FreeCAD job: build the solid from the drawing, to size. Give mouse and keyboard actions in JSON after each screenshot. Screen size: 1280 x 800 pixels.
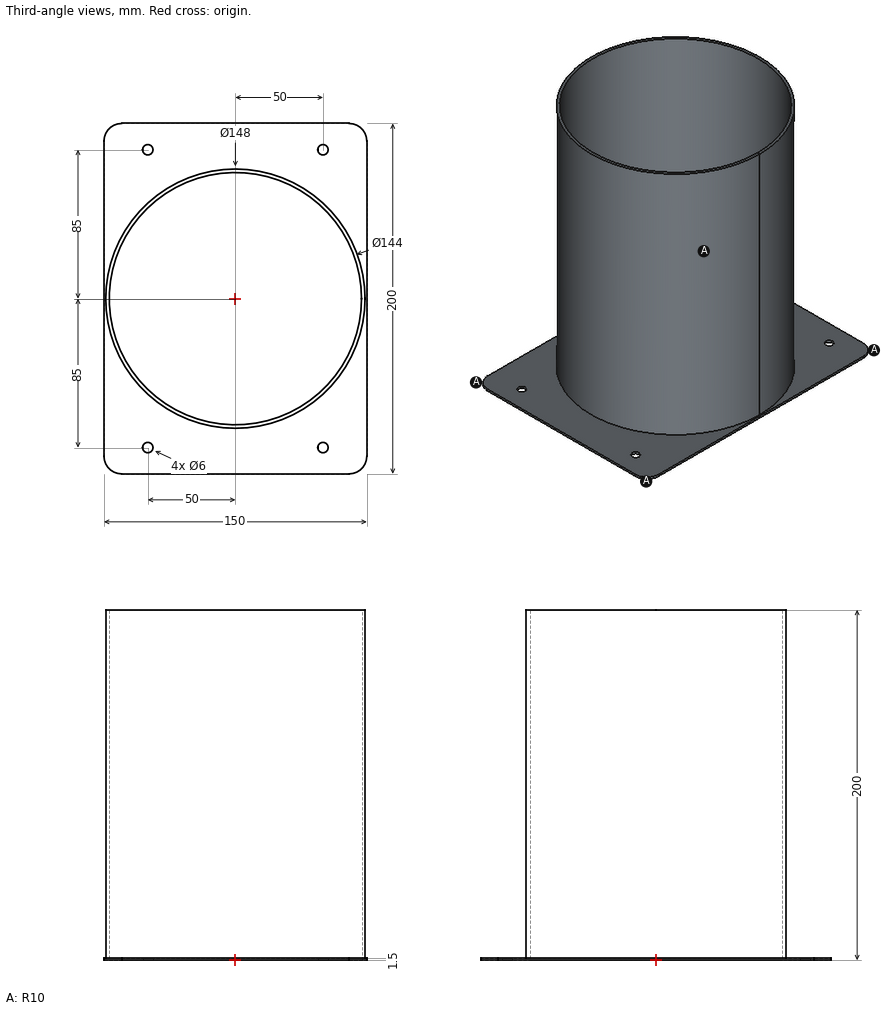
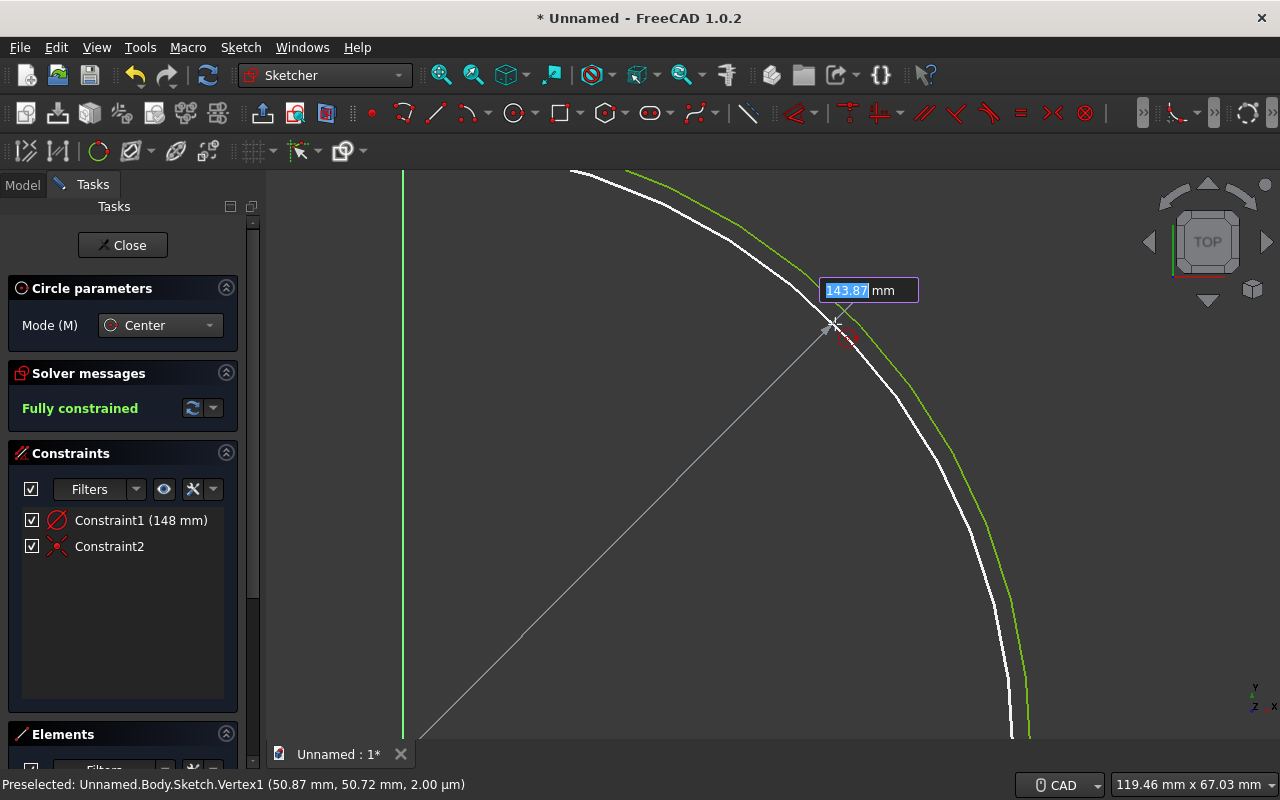
{"action": "type", "text": "144"}
{"action": "key", "text": "Return"}
{"action": "key", "text": "Escape"}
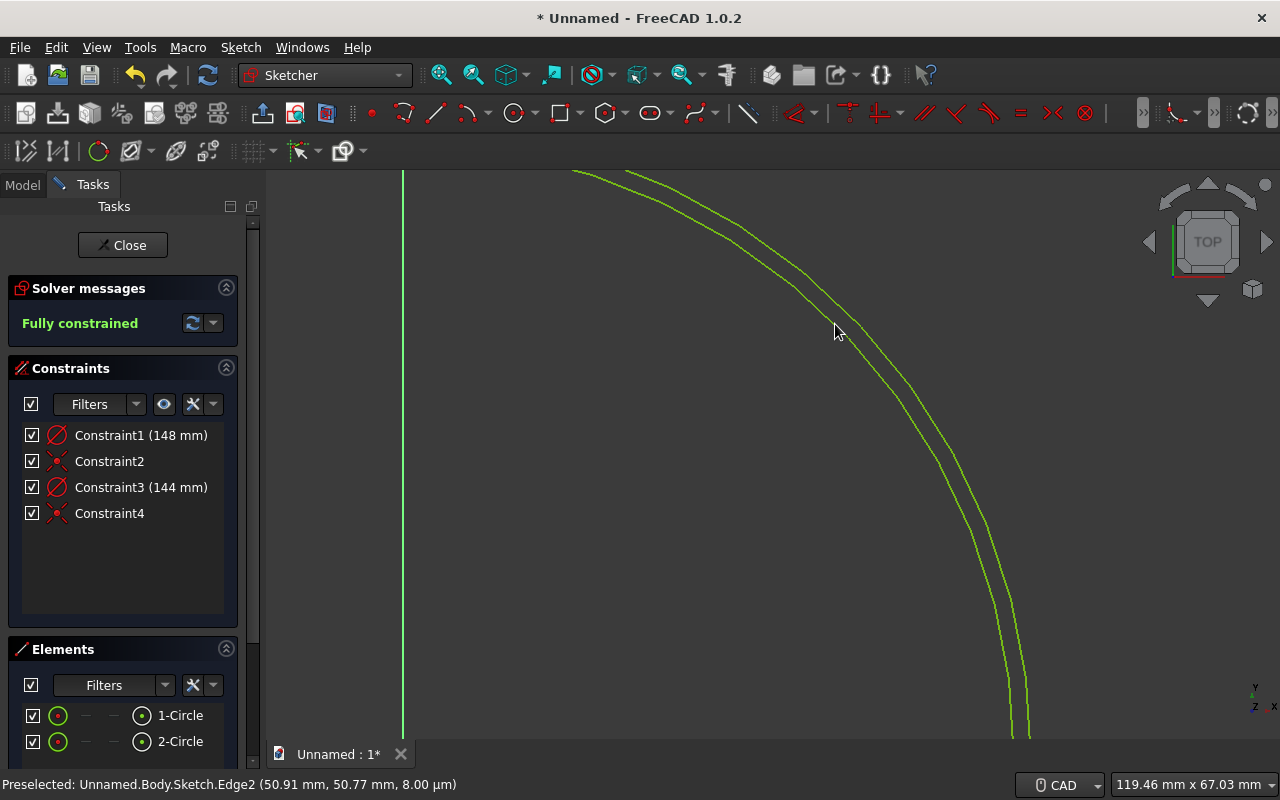
{"action": "left_click", "coordinate": [123, 245]}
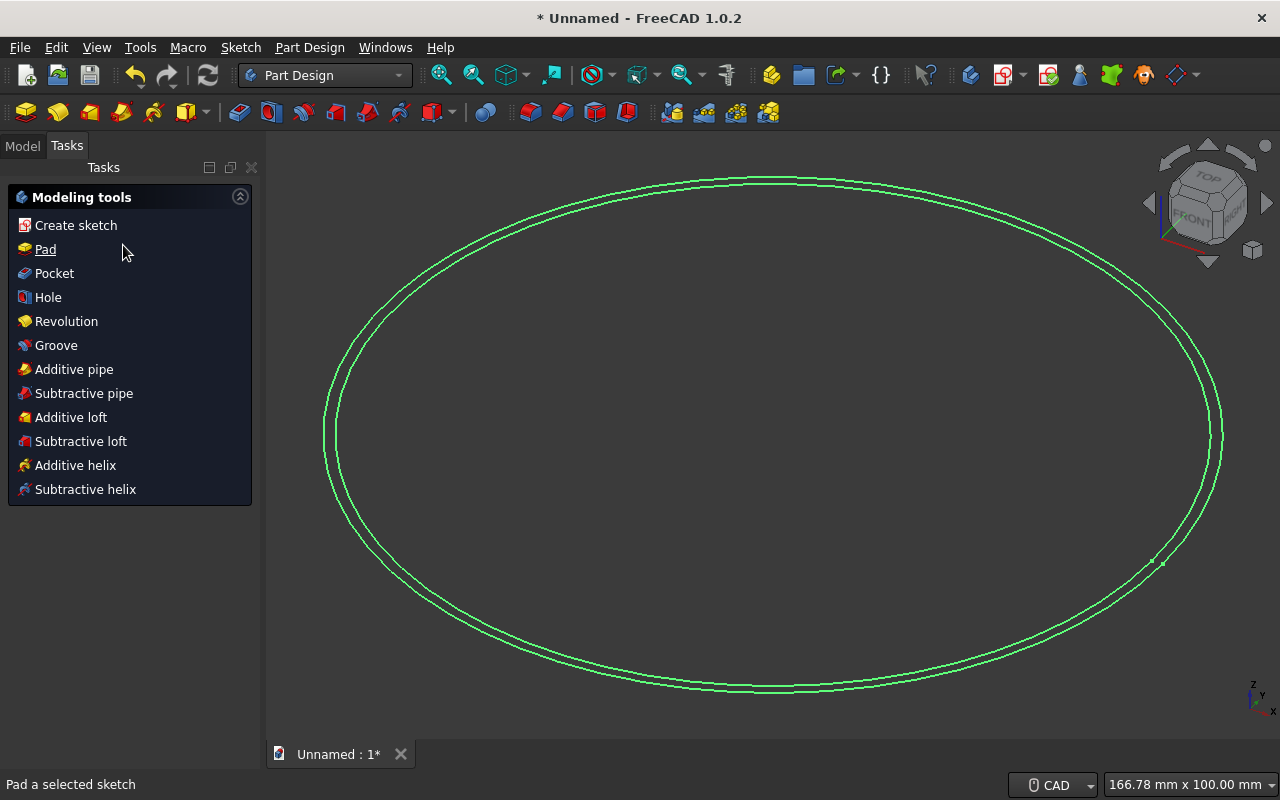
{"action": "left_click", "coordinate": [26, 112]}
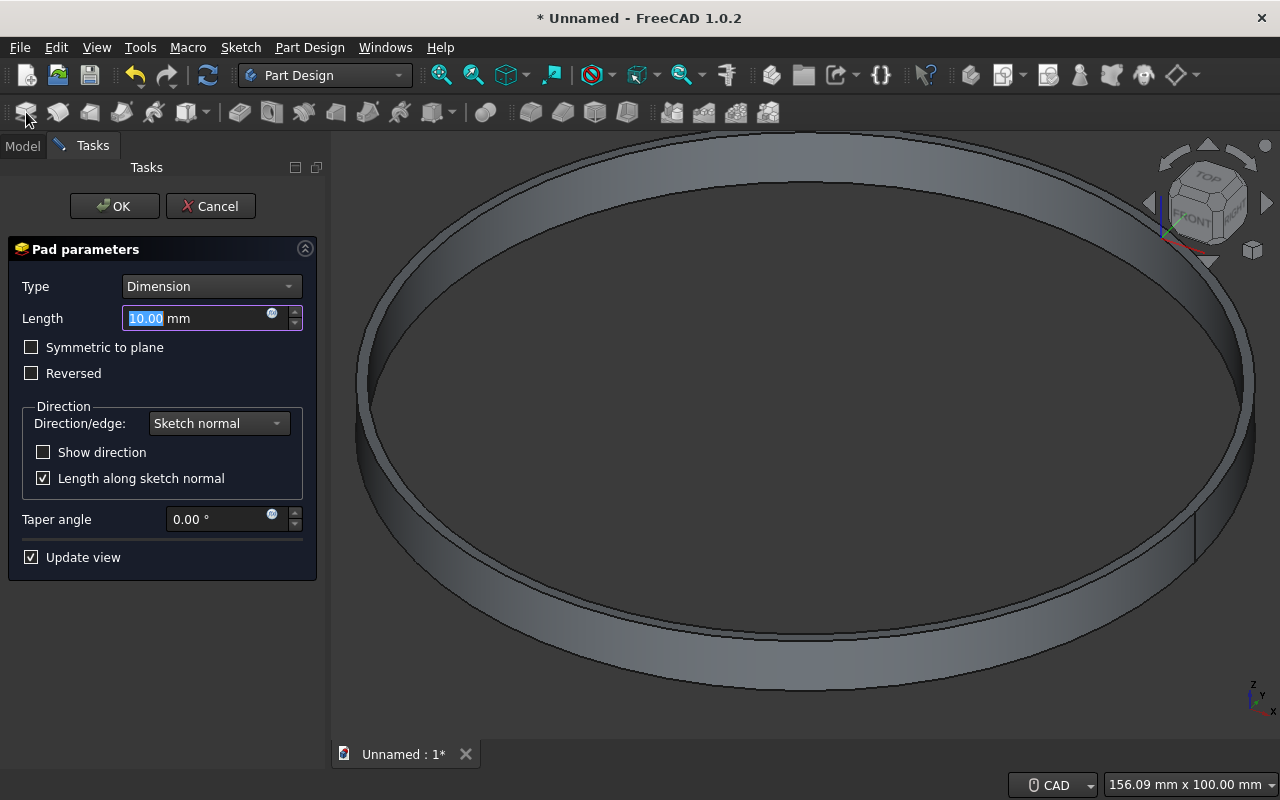
{"action": "type", "text": "200"}
{"action": "key", "text": "Tab"}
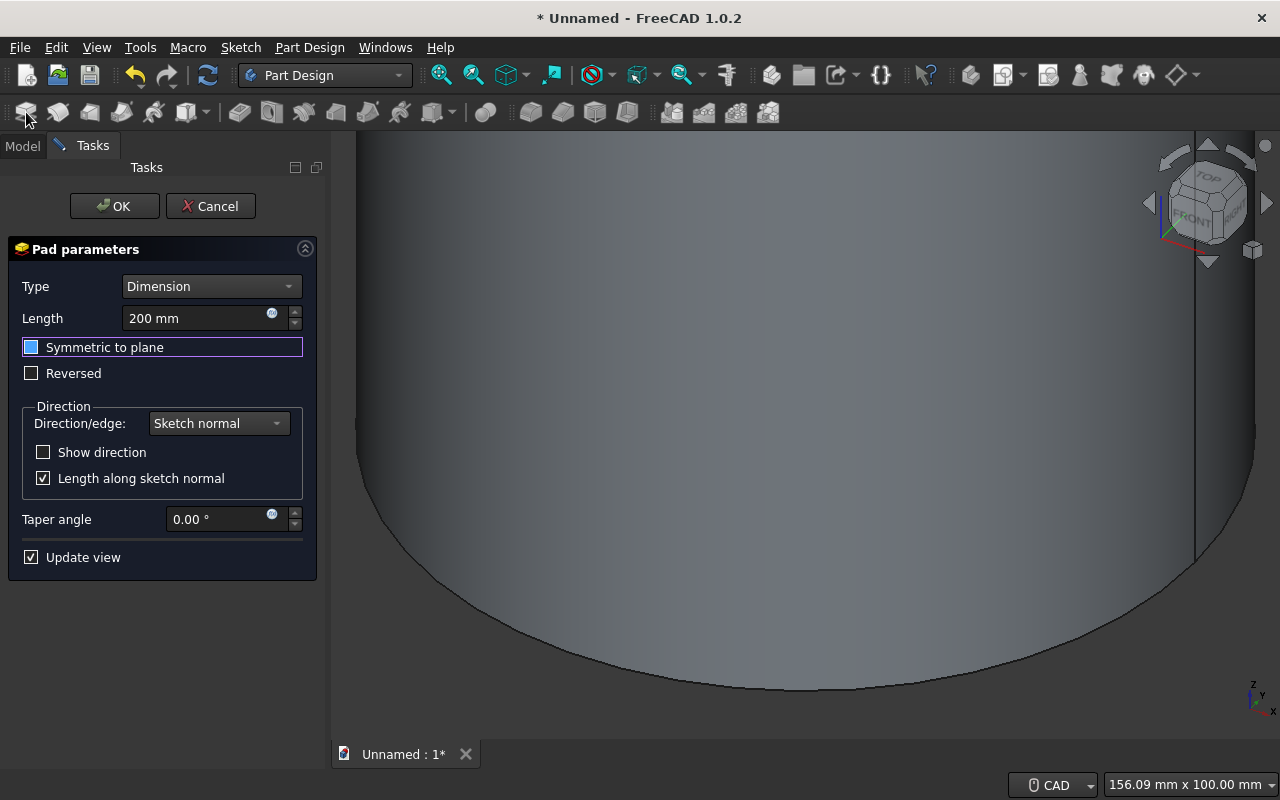
{"action": "left_click", "coordinate": [115, 206]}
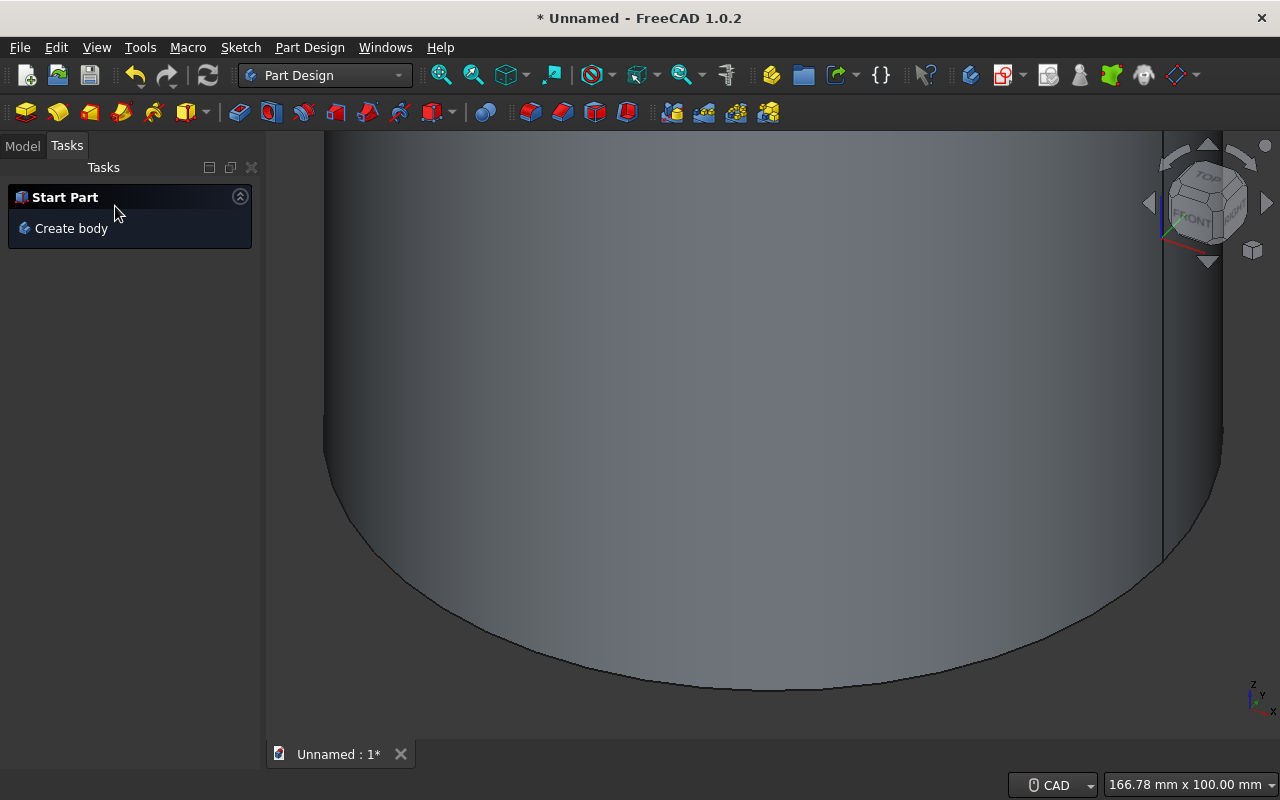
{"action": "left_click", "coordinate": [442, 76]}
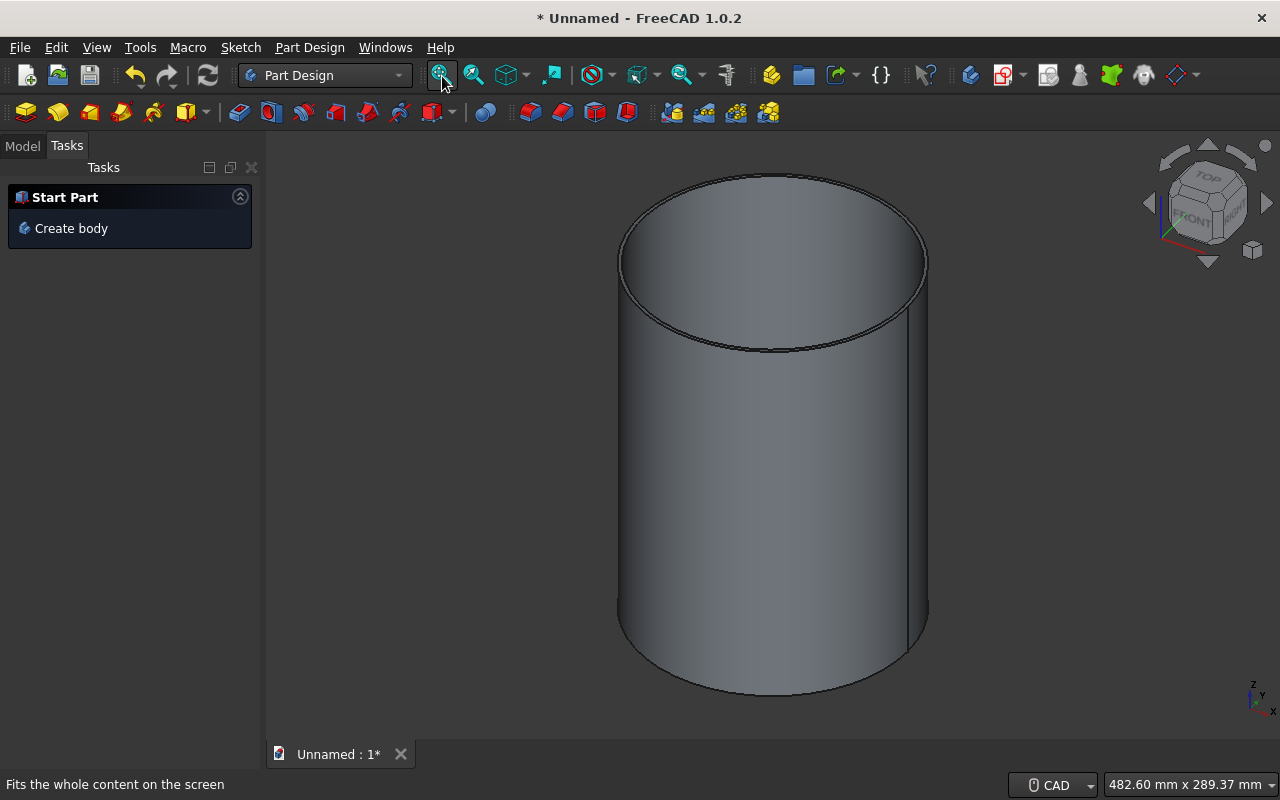
{"action": "left_click", "coordinate": [1004, 76]}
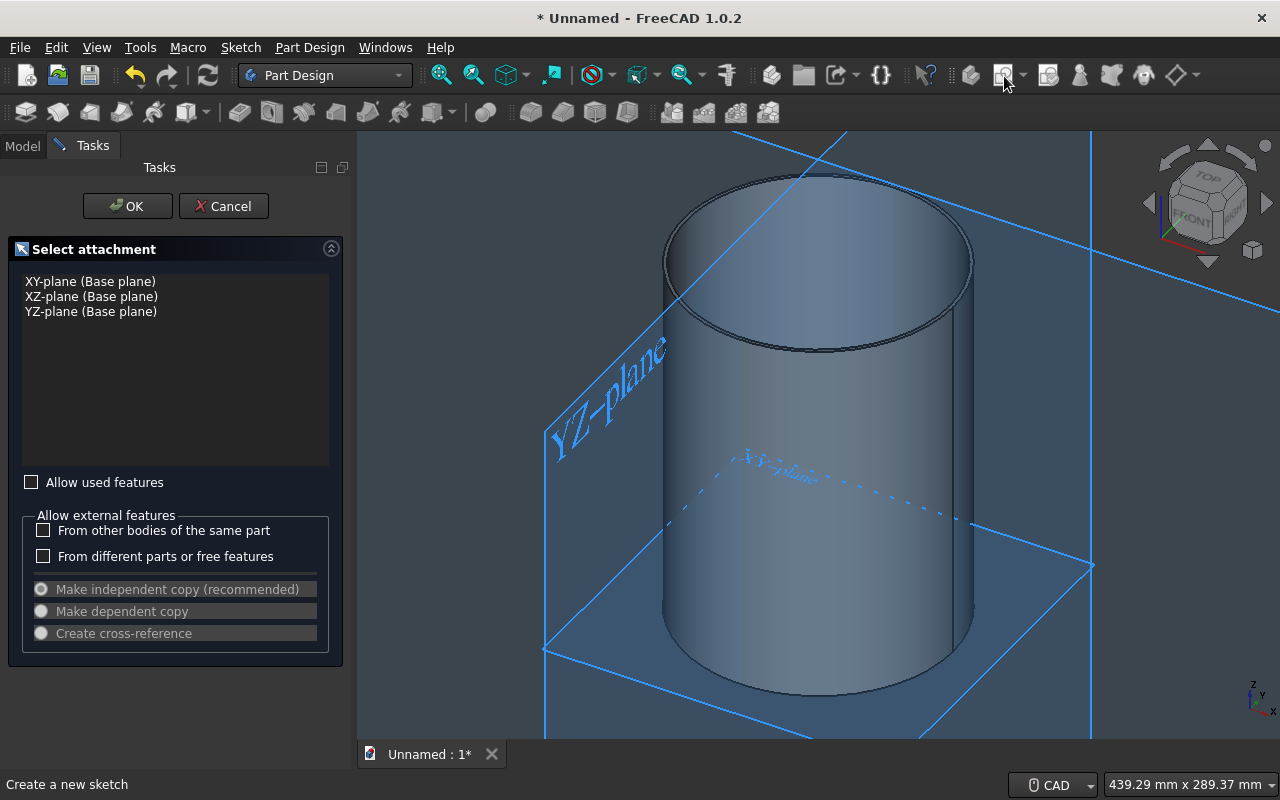
{"action": "left_click", "coordinate": [82, 282]}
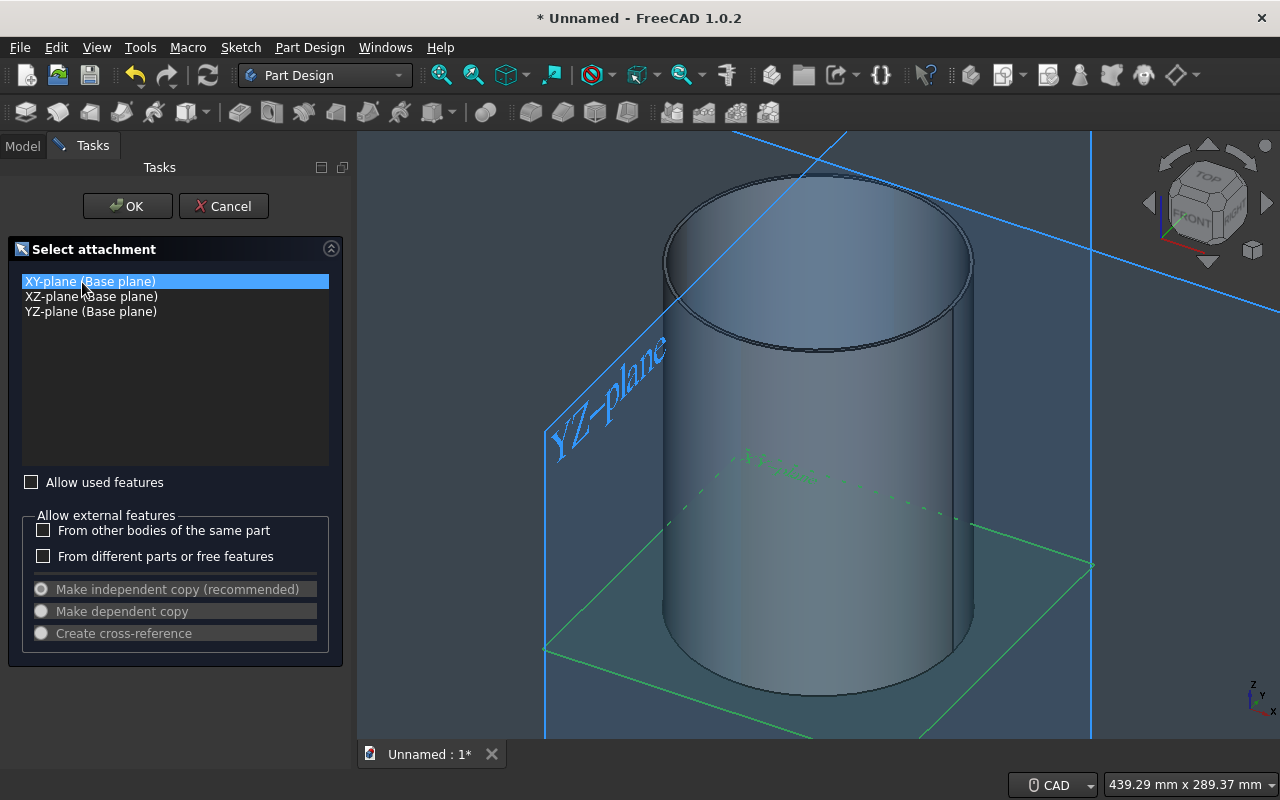
{"action": "left_click", "coordinate": [128, 206]}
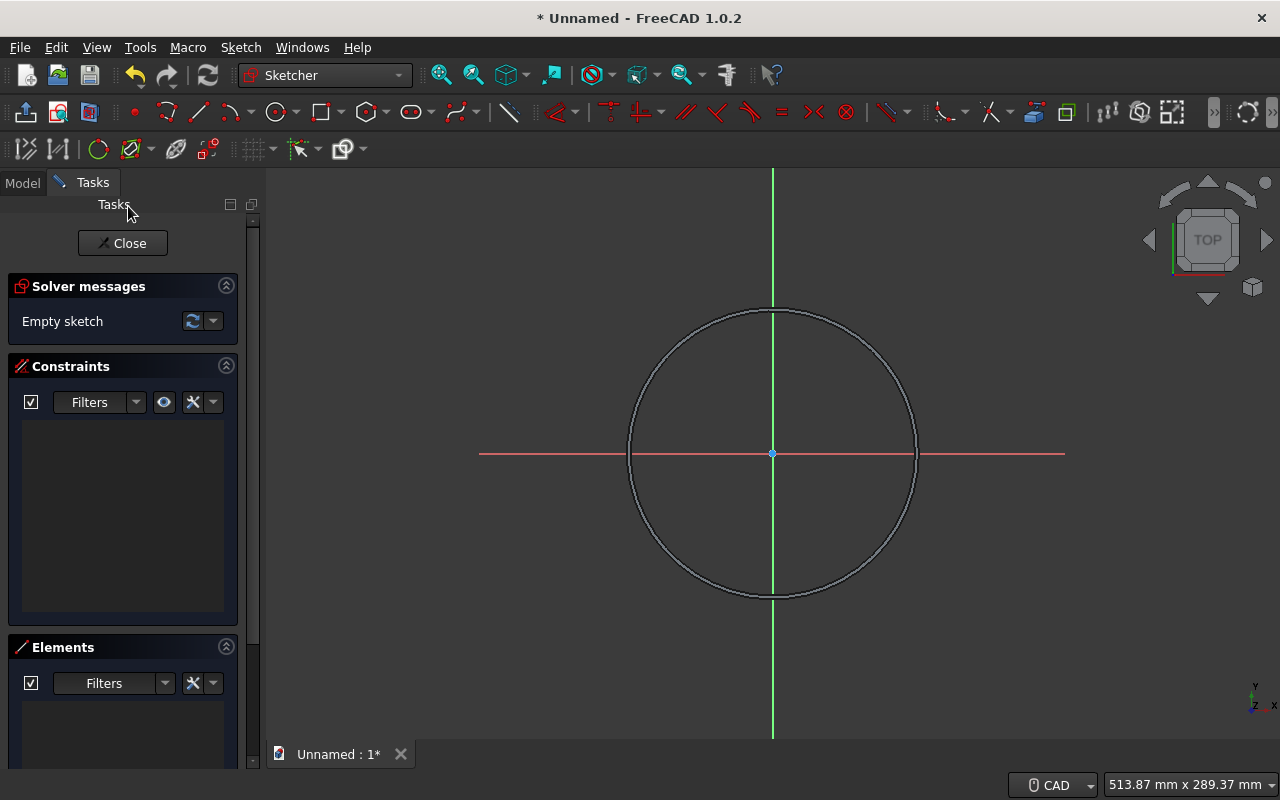
{"action": "left_click", "coordinate": [90, 112]}